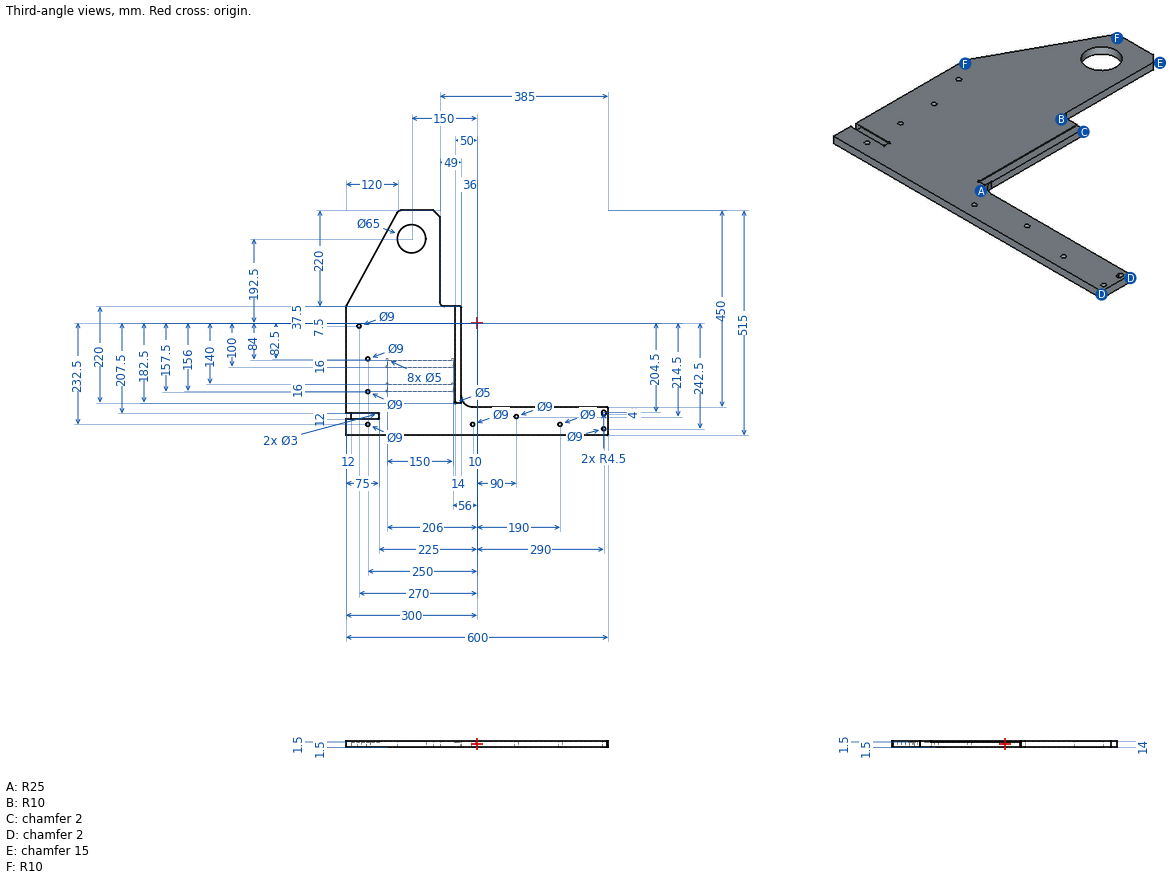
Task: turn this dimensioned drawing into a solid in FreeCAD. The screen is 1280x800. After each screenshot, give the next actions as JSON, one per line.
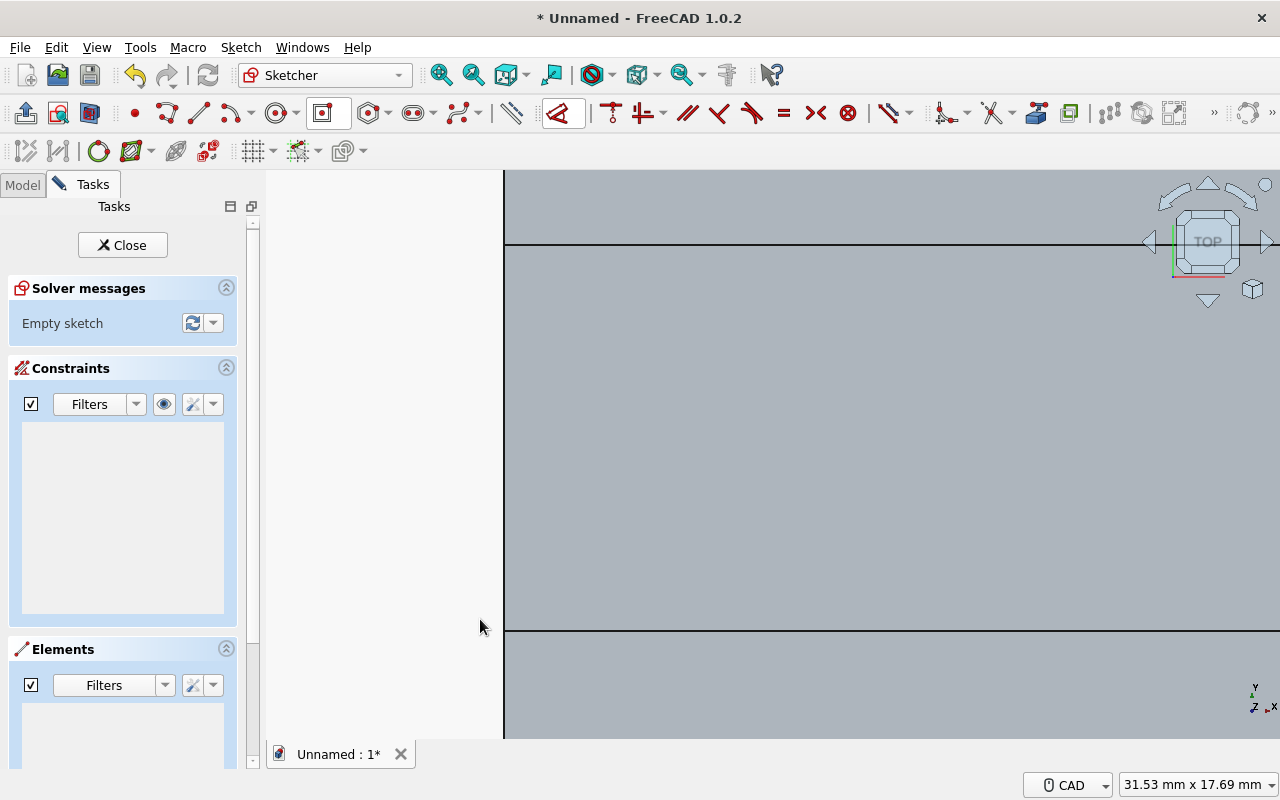
{"action": "left_click", "coordinate": [346, 114]}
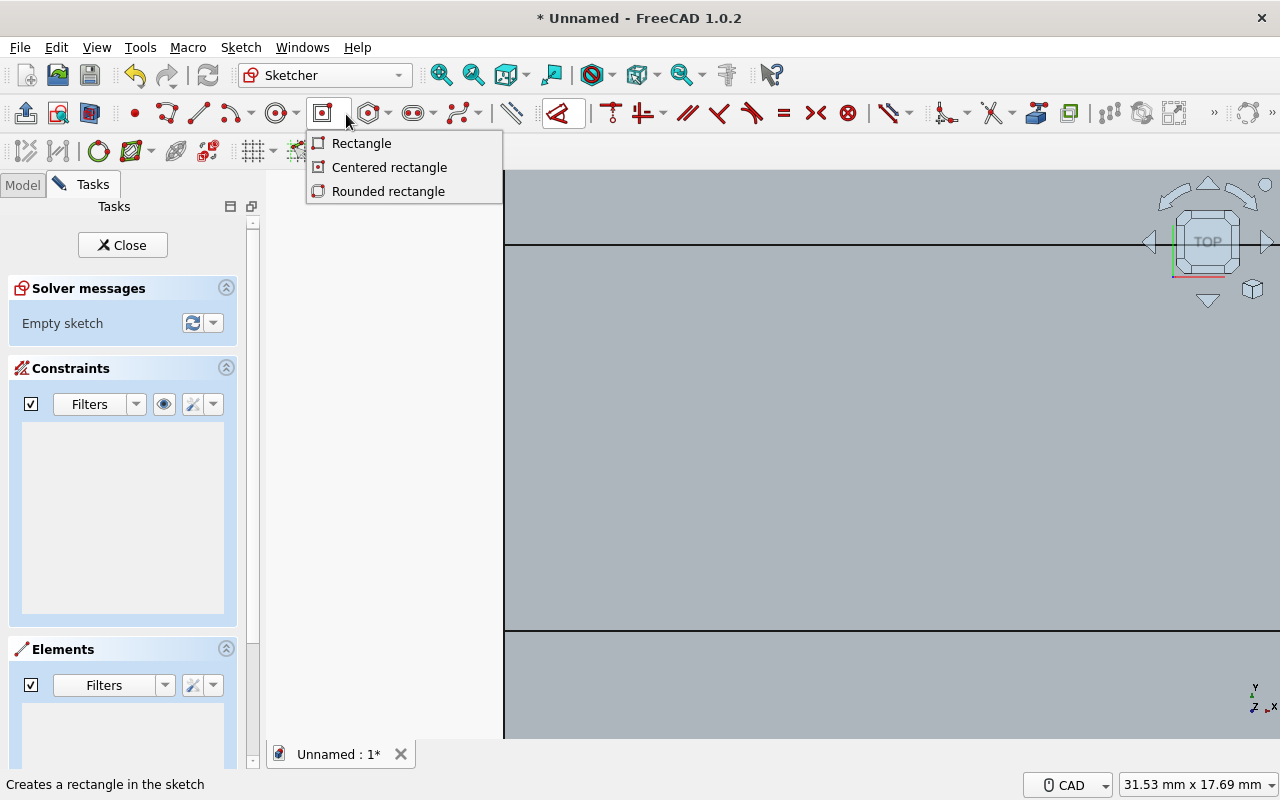
{"action": "left_click", "coordinate": [404, 143]}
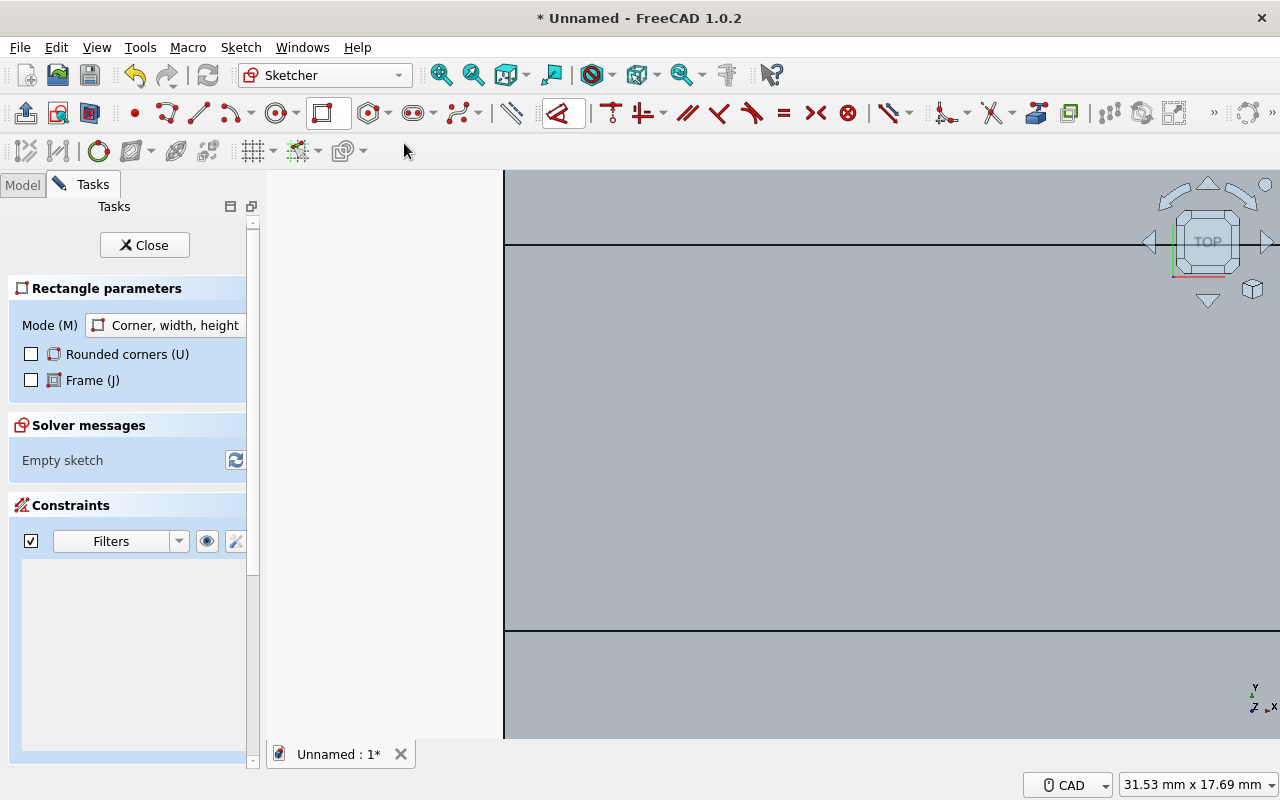
{"action": "left_click", "coordinate": [504, 245]}
{"action": "mouse_move", "coordinate": [890, 631]}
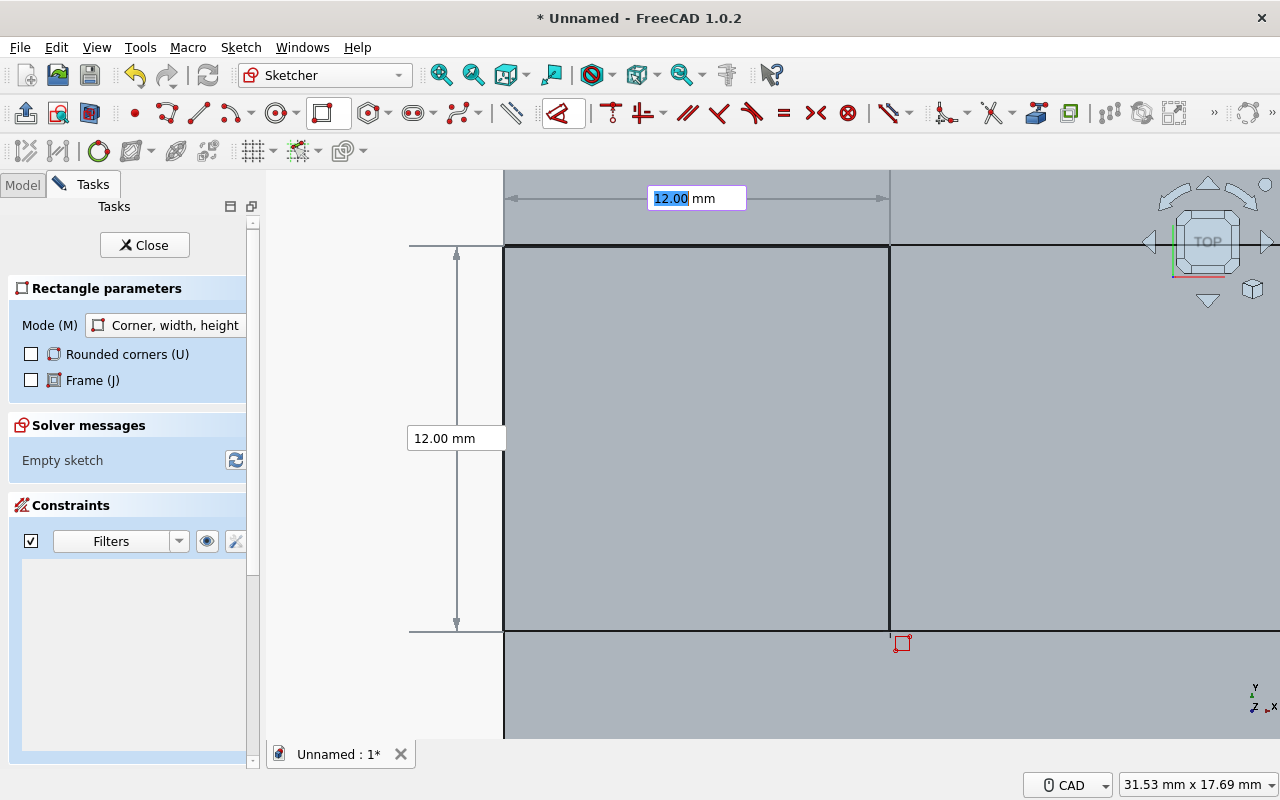
{"action": "type", "text": "12"}
{"action": "key", "text": "Tab"}
{"action": "type", "text": "12"}
{"action": "key", "text": "Return"}
{"action": "key", "text": "Escape"}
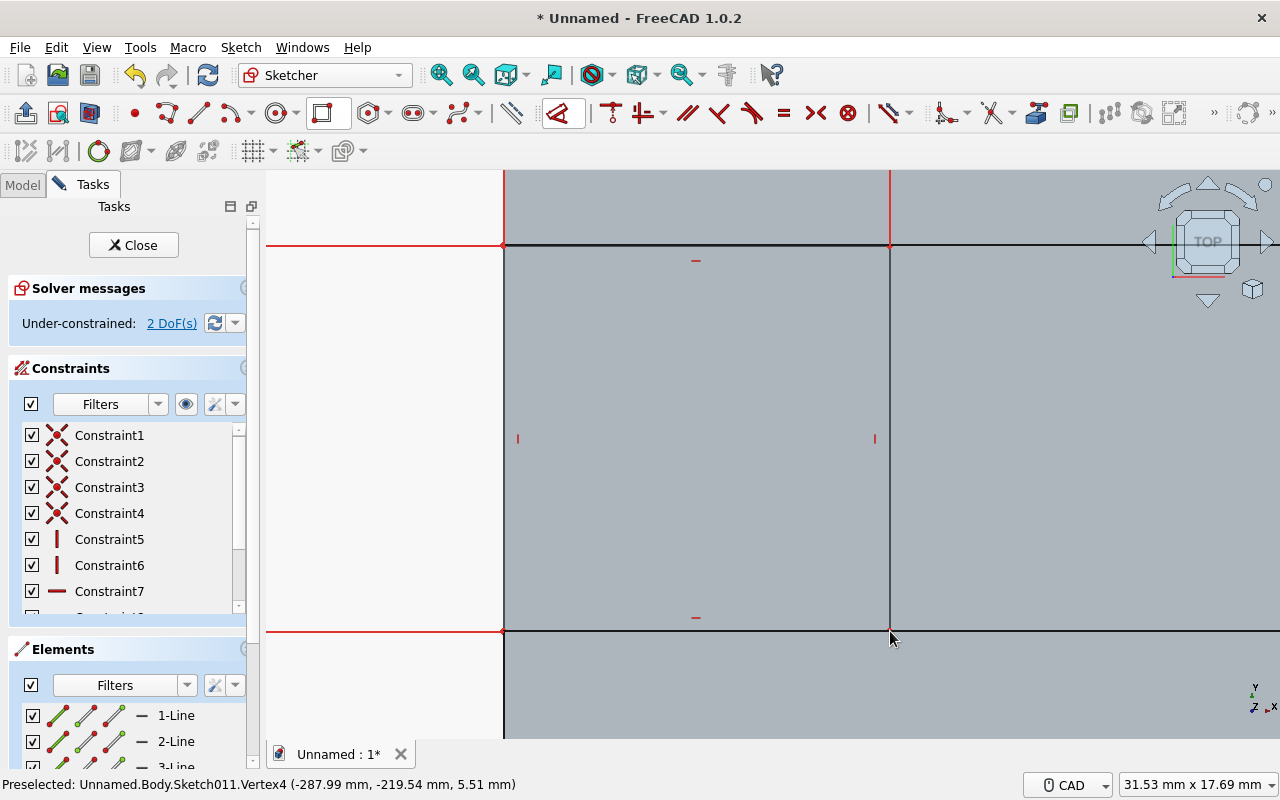
{"action": "left_click", "coordinate": [504, 246]}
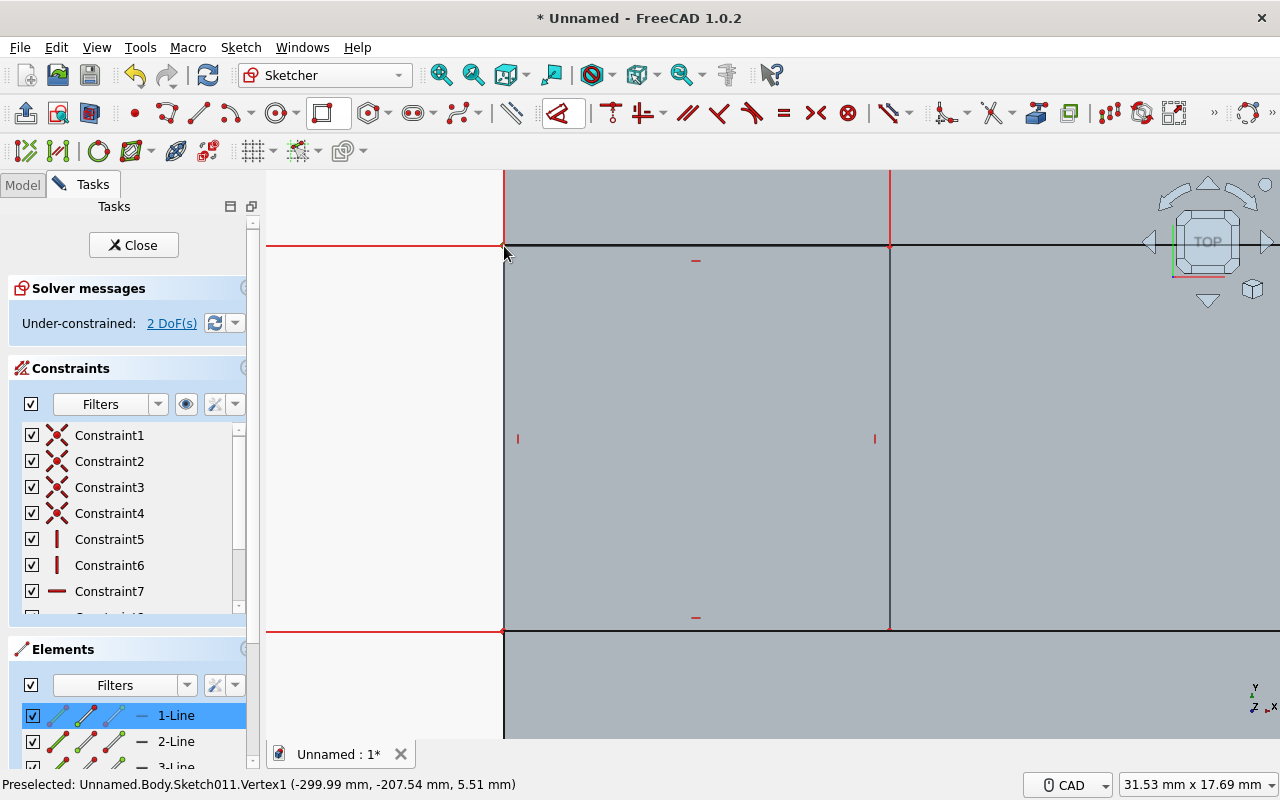
{"action": "left_click", "coordinate": [580, 114]}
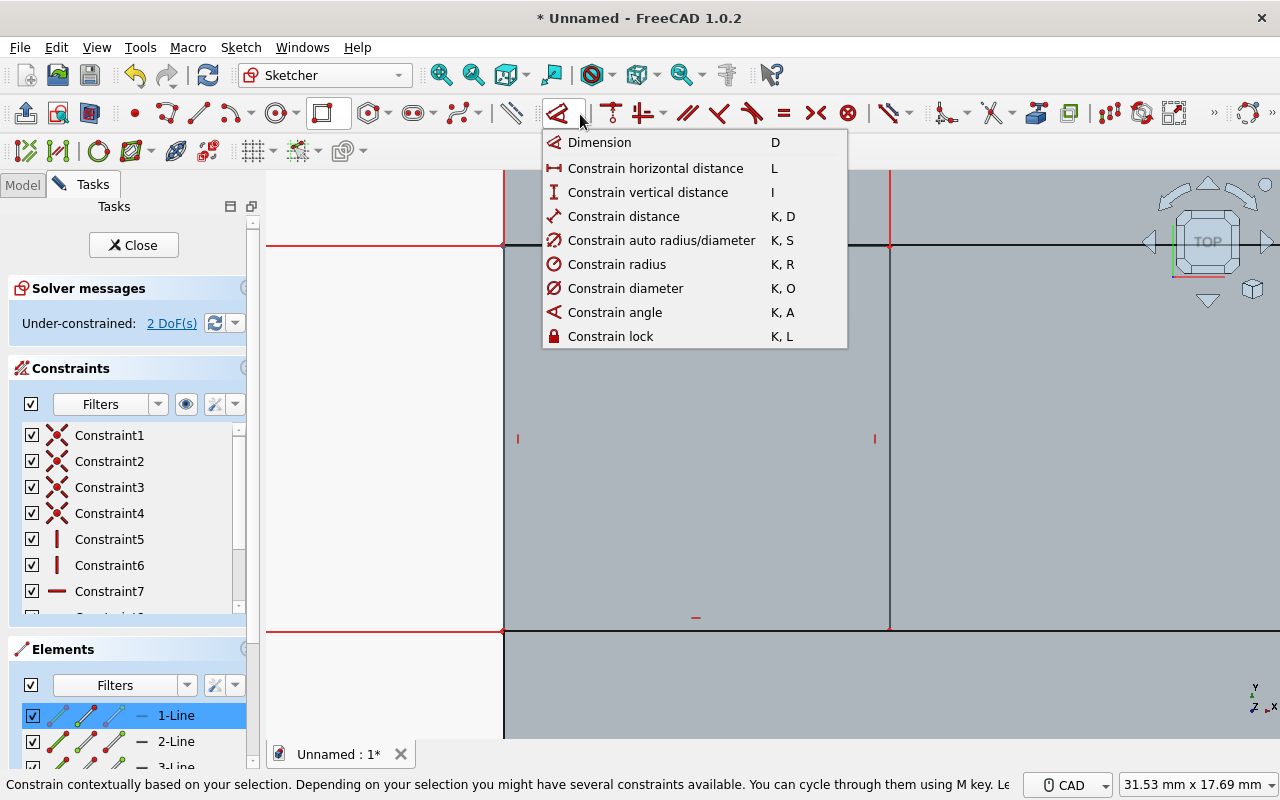
{"action": "left_click", "coordinate": [695, 168]}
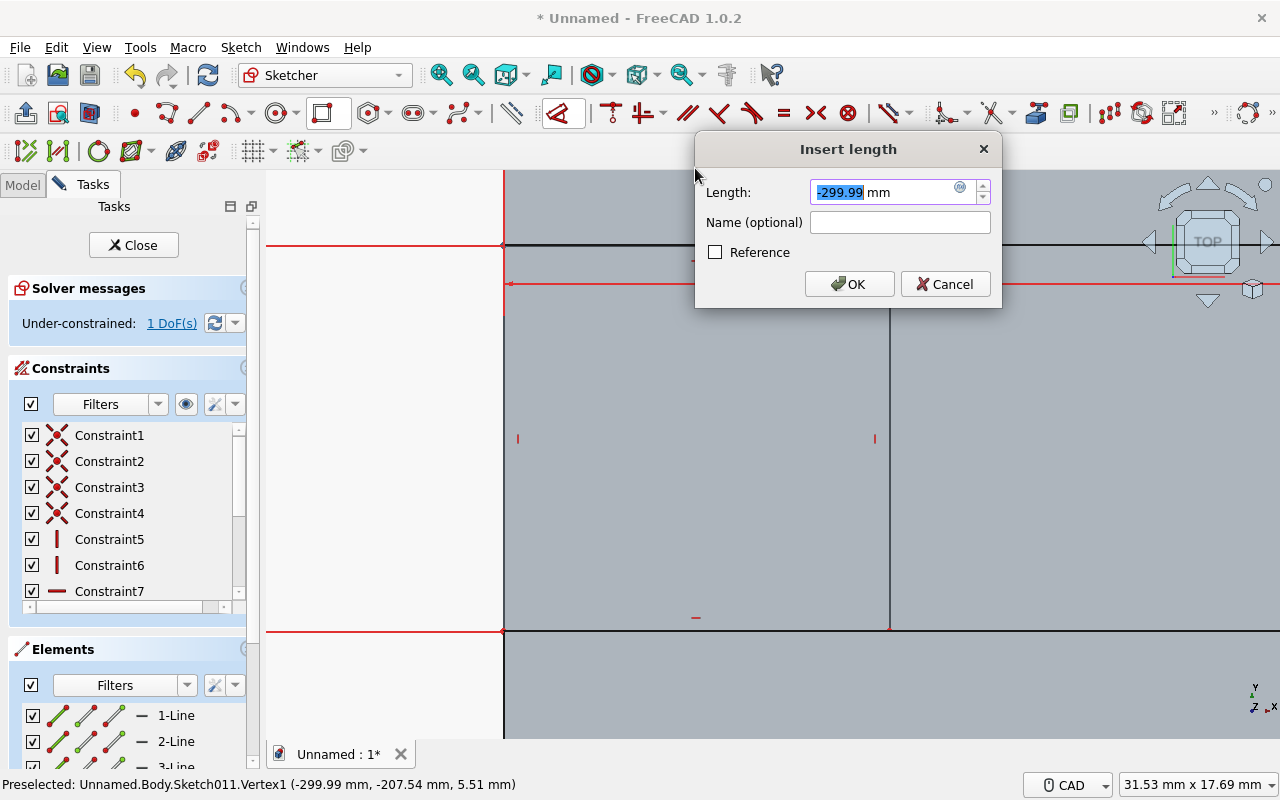
{"action": "type", "text": "-300"}
{"action": "key", "text": "Return"}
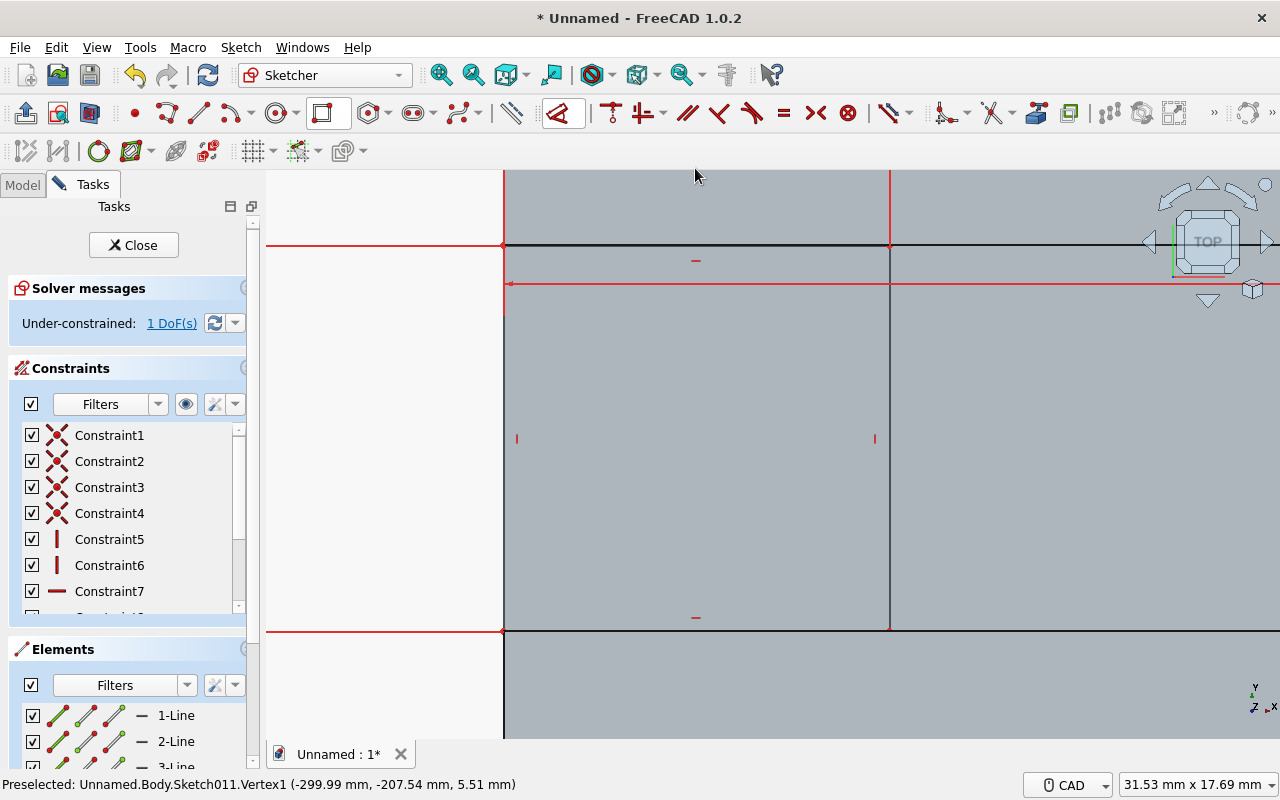
{"action": "left_click", "coordinate": [504, 246]}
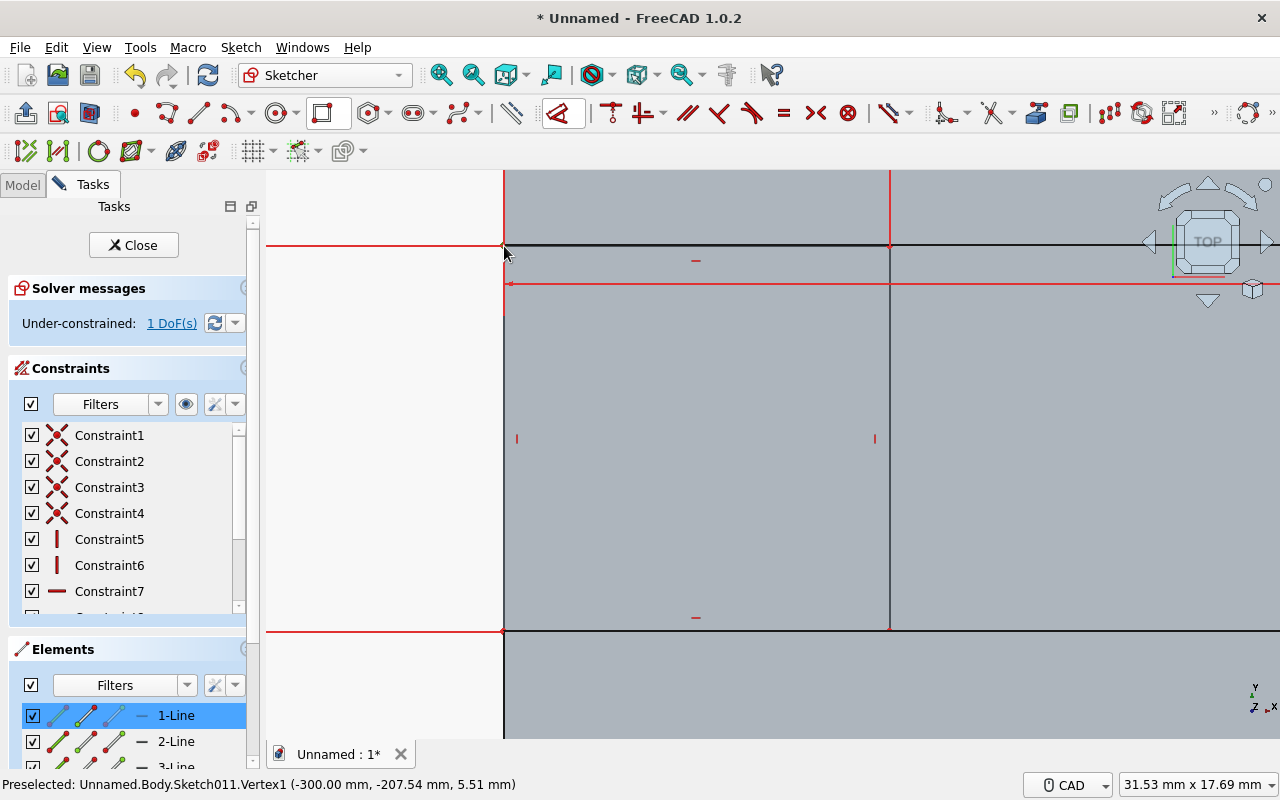
{"action": "left_click", "coordinate": [580, 114]}